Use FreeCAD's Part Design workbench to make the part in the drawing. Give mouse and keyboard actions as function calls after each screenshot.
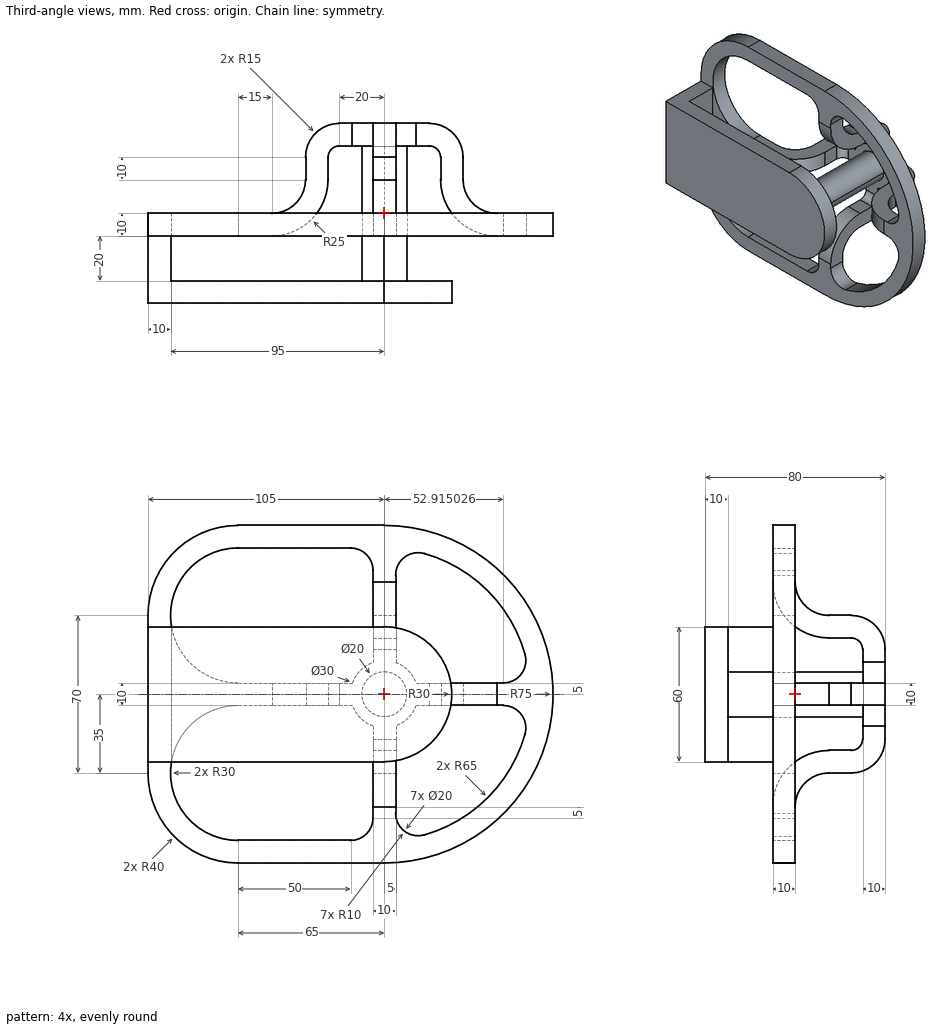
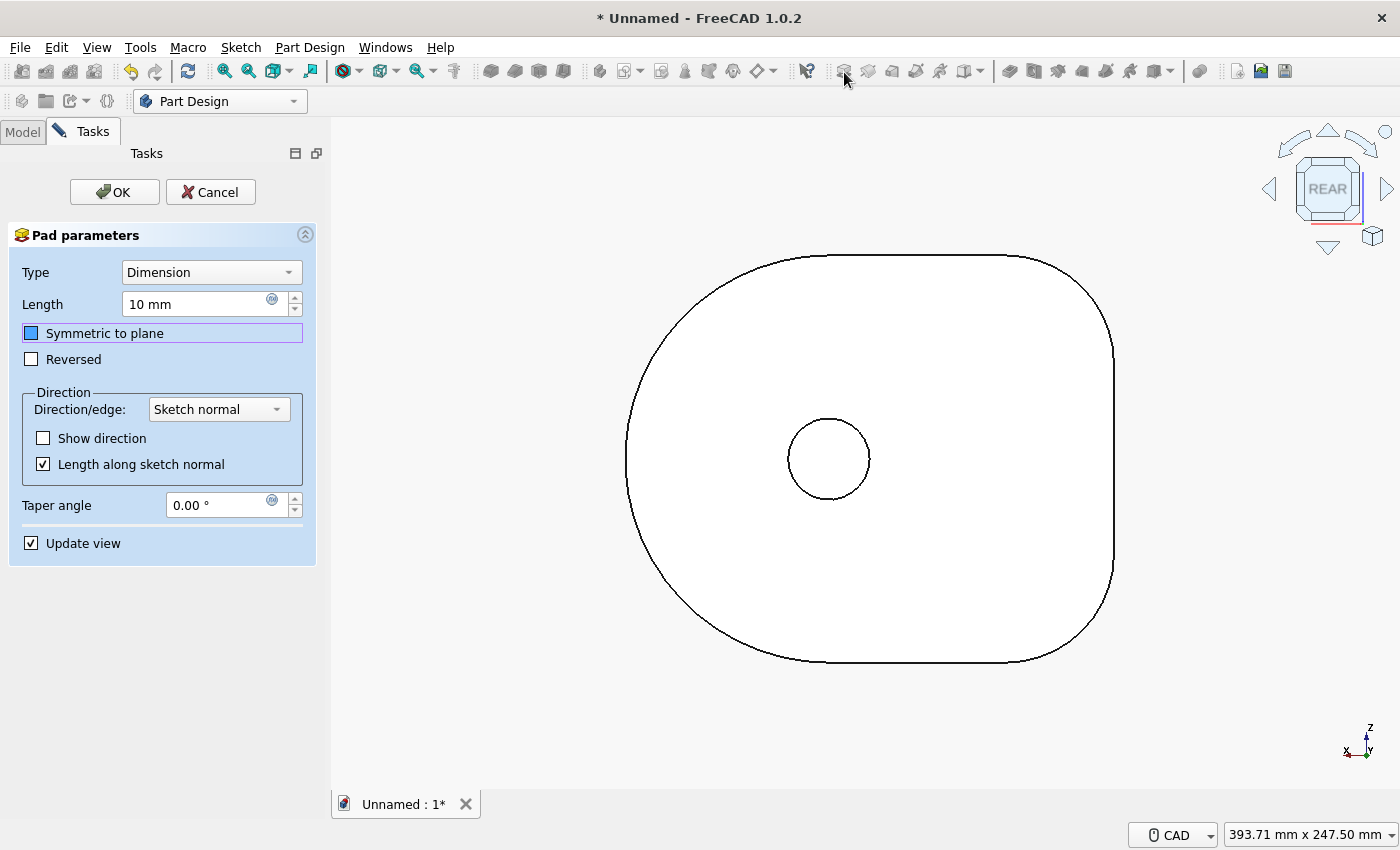
click(30, 359)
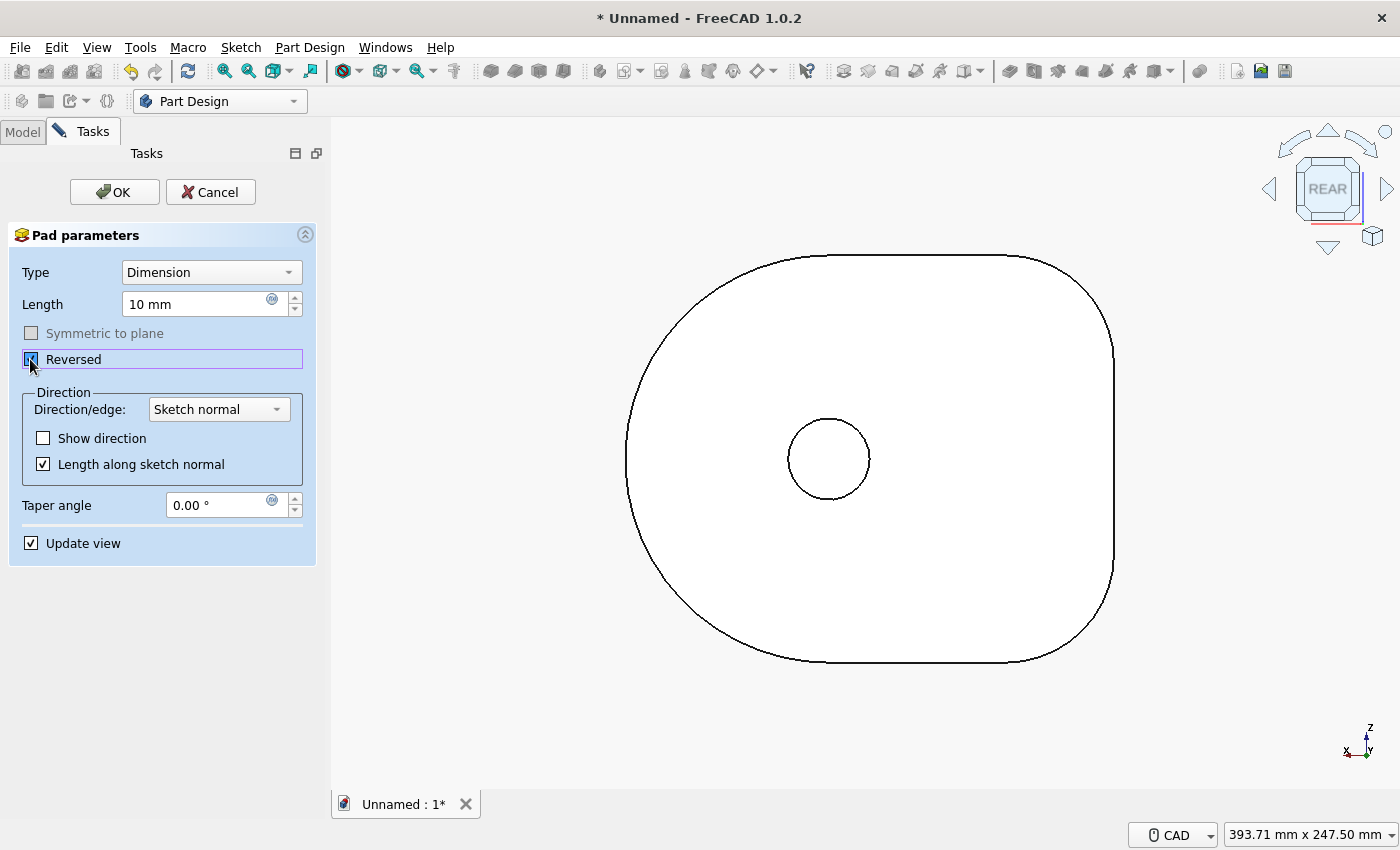
click(115, 192)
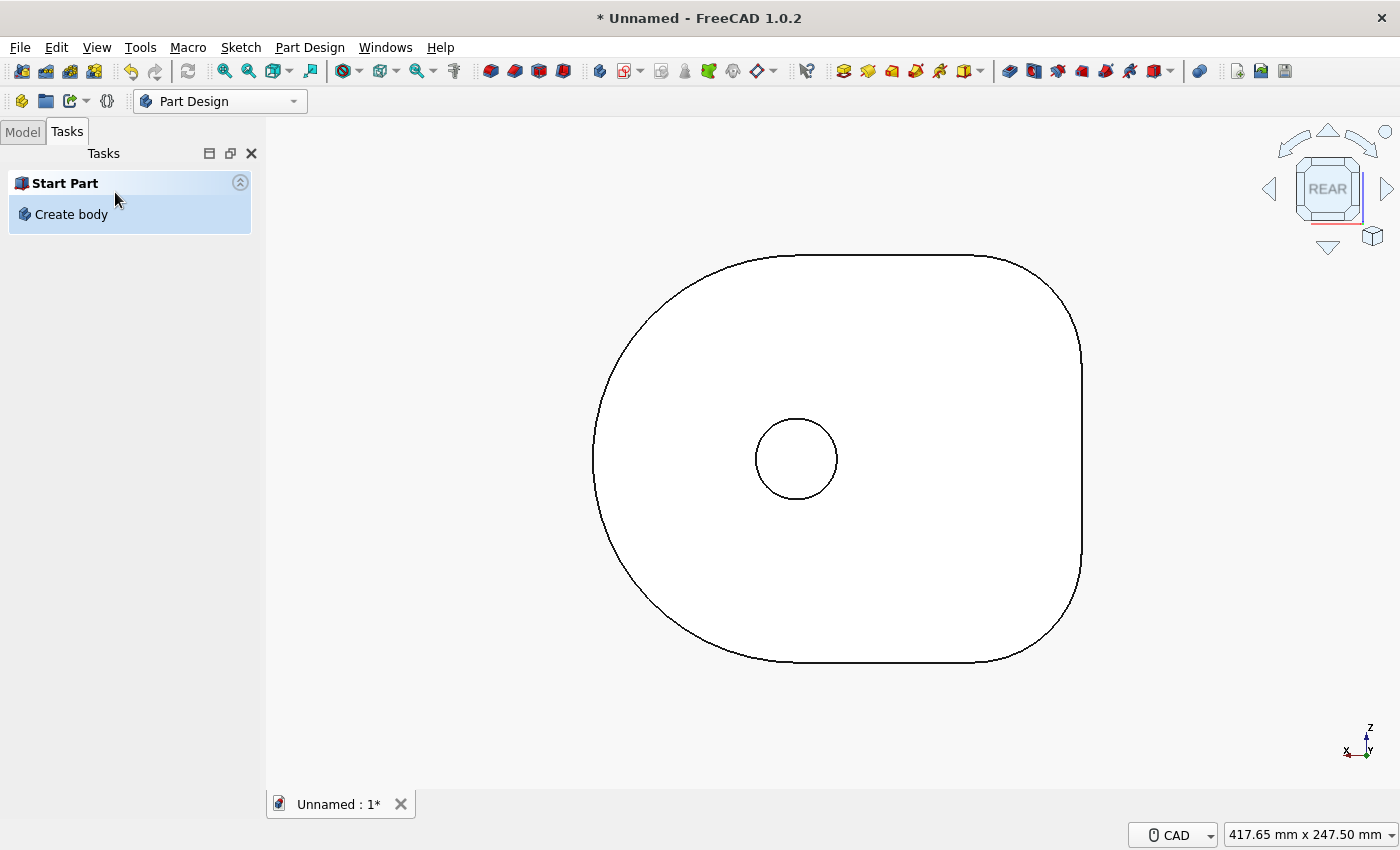
click(624, 72)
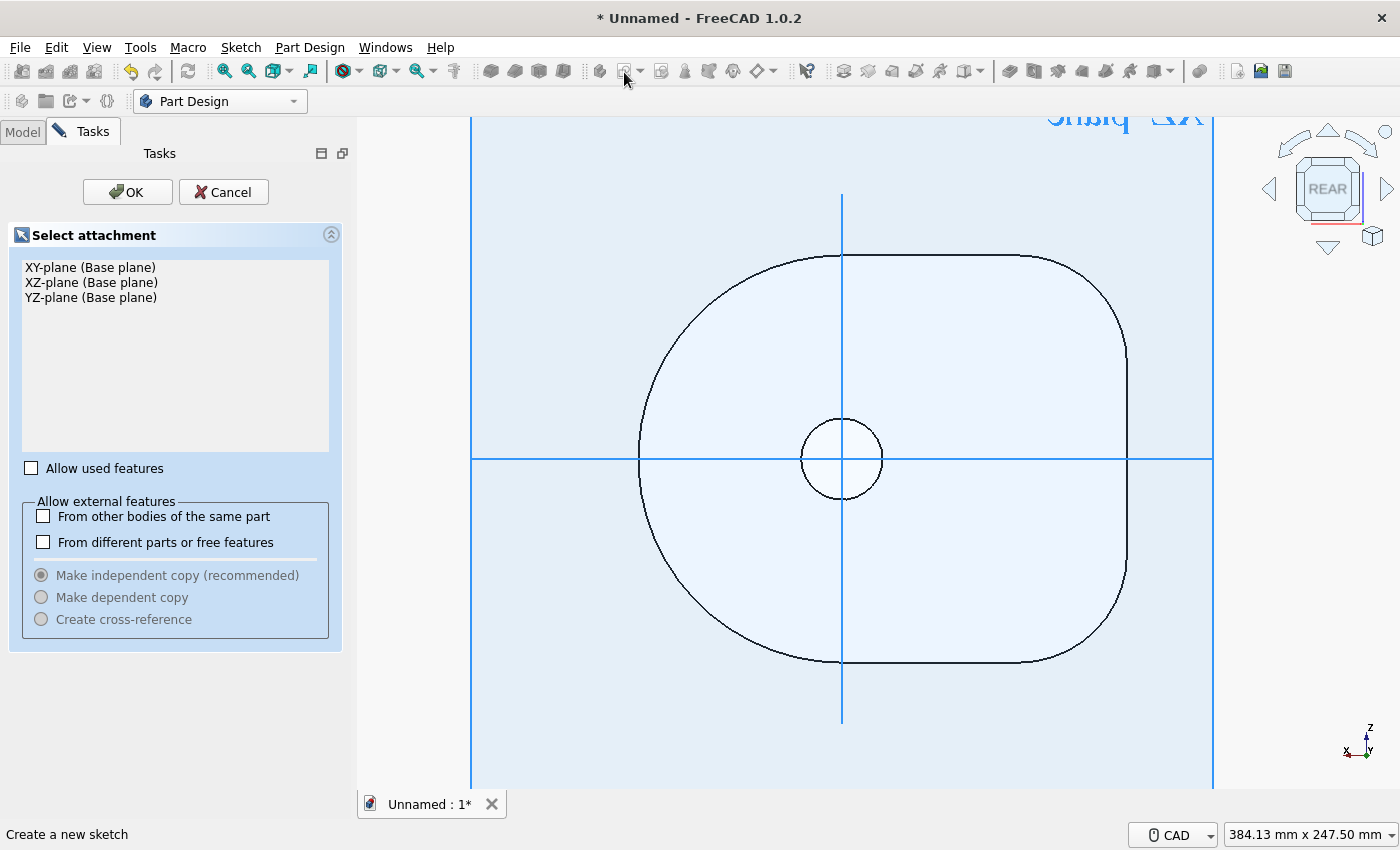
click(82, 282)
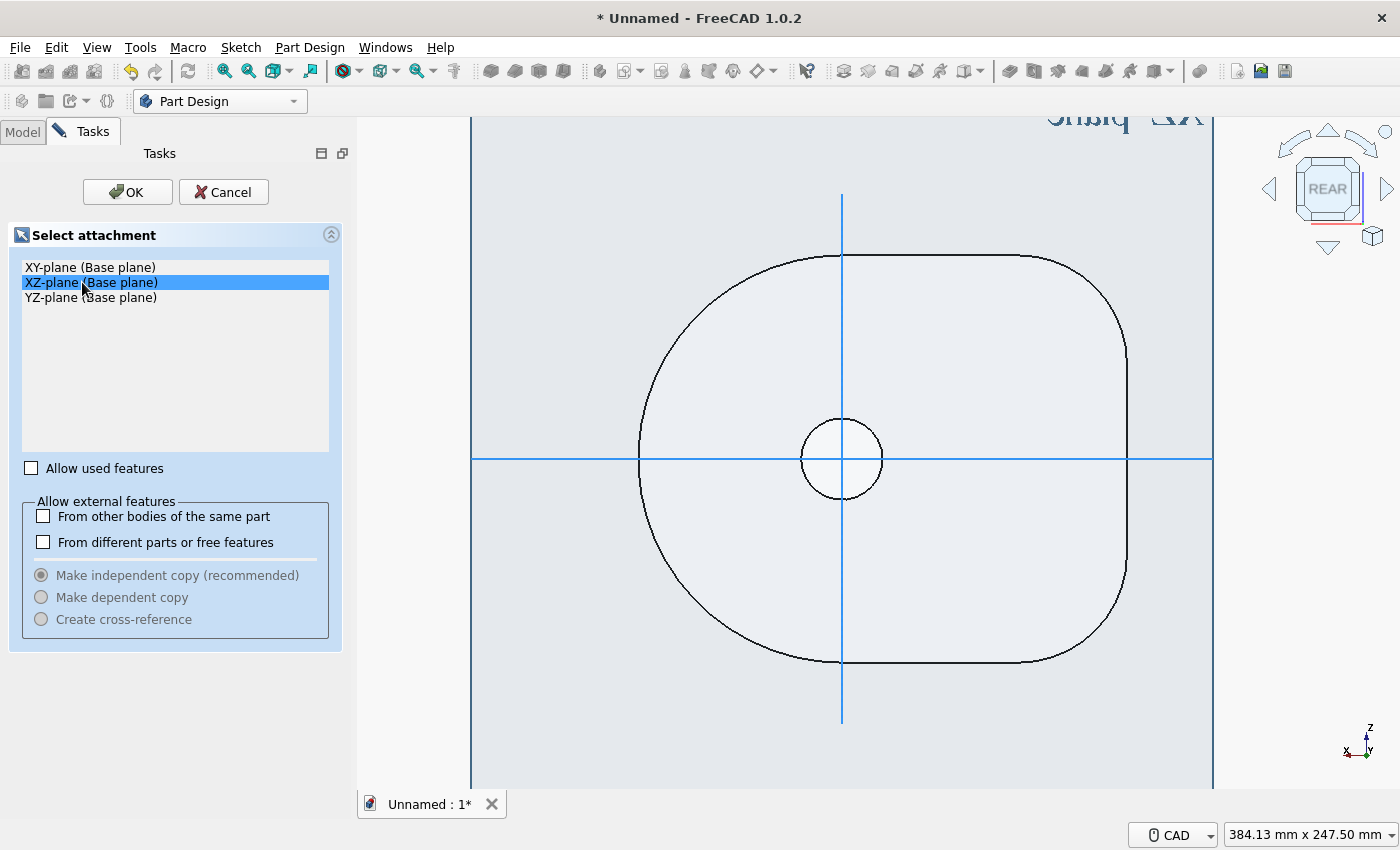
click(128, 192)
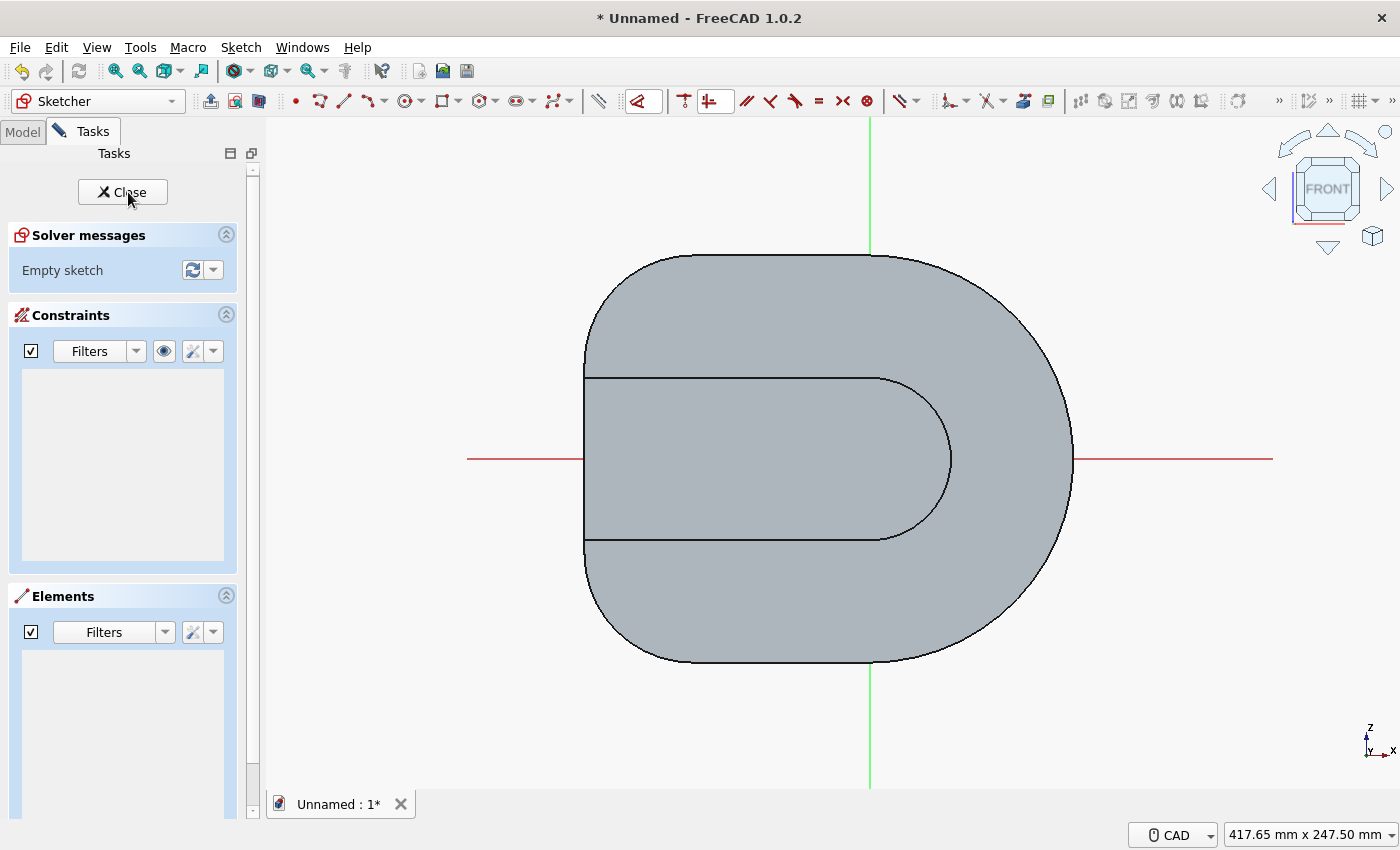
click(260, 102)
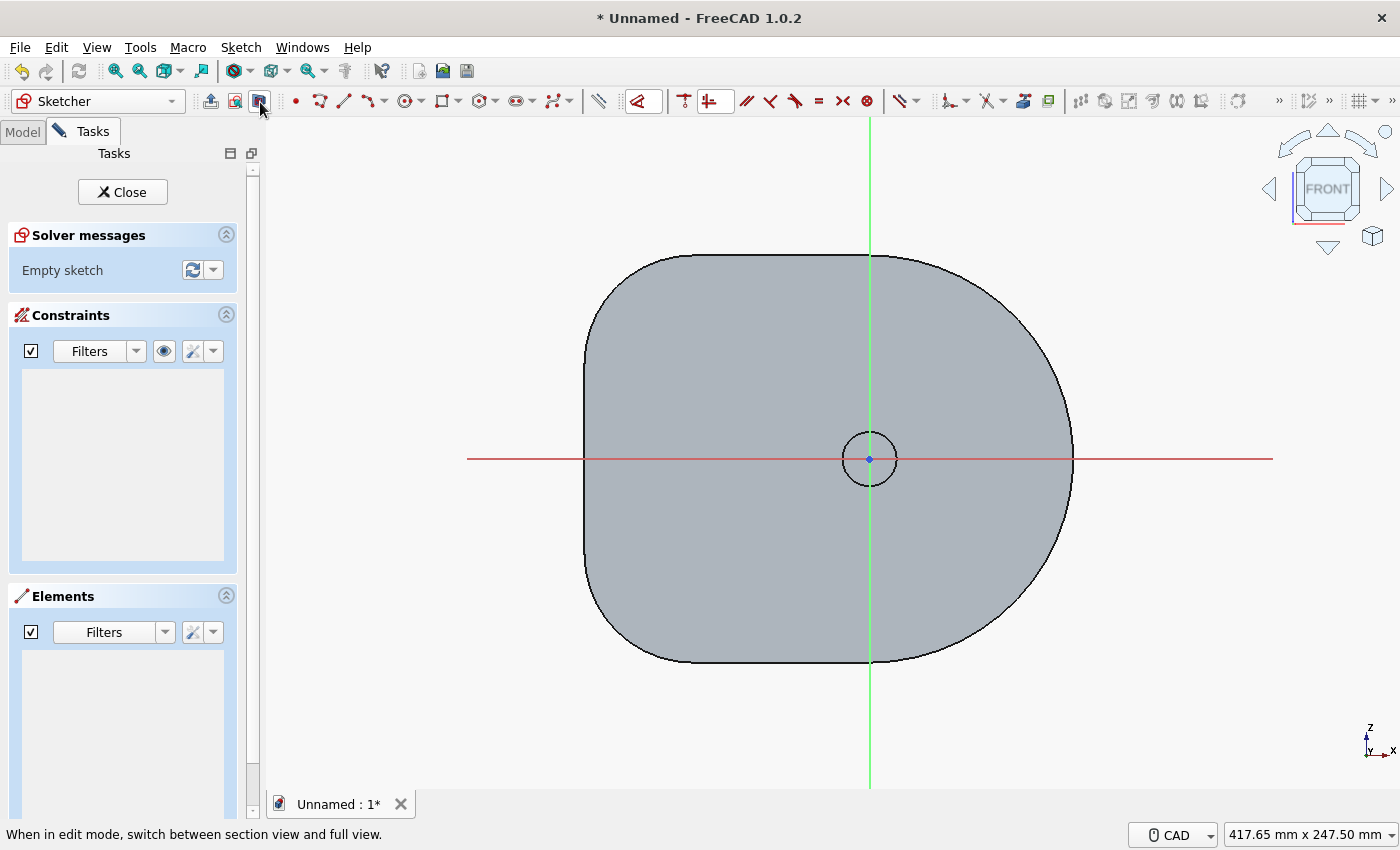
click(320, 102)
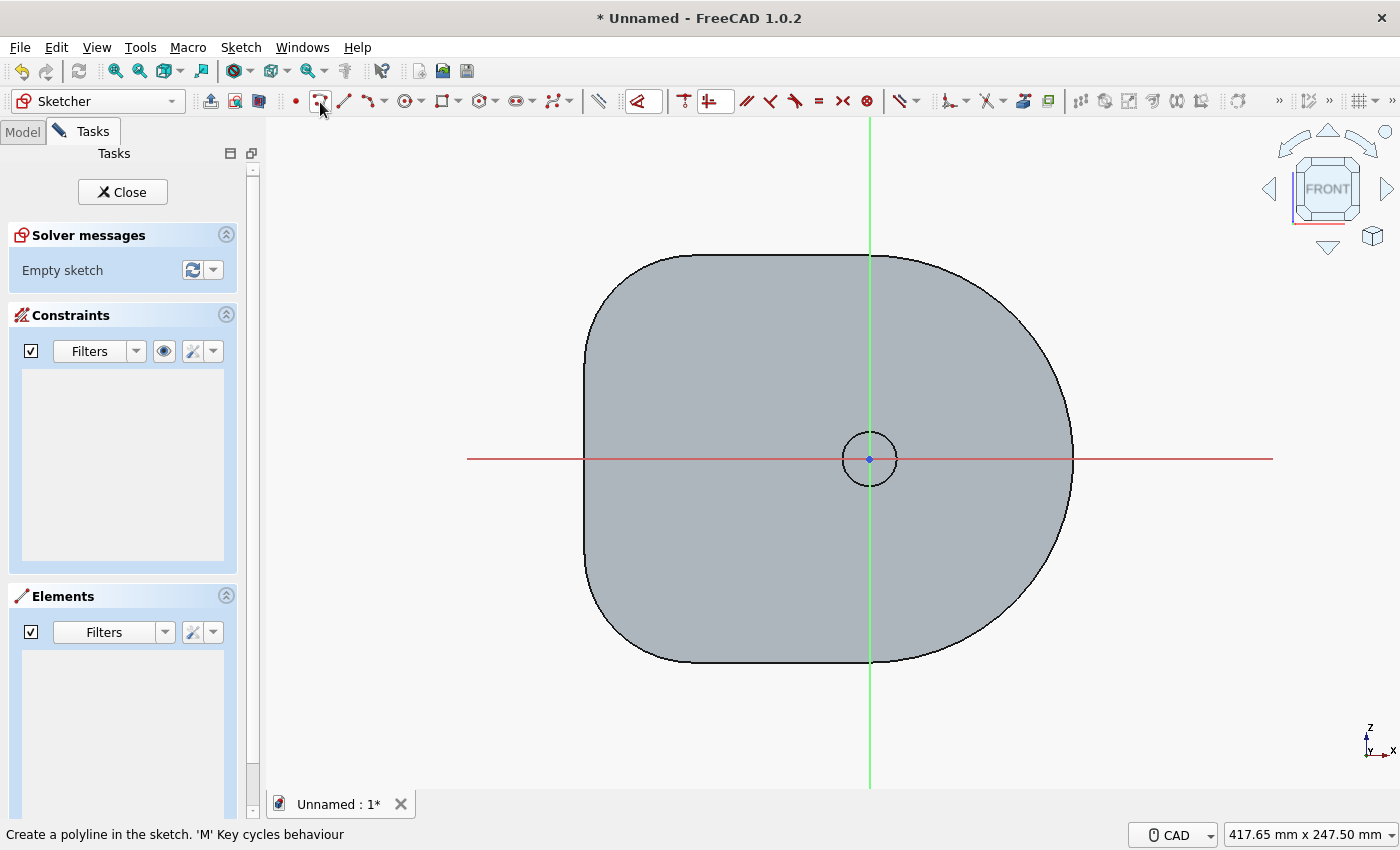
click(883, 603)